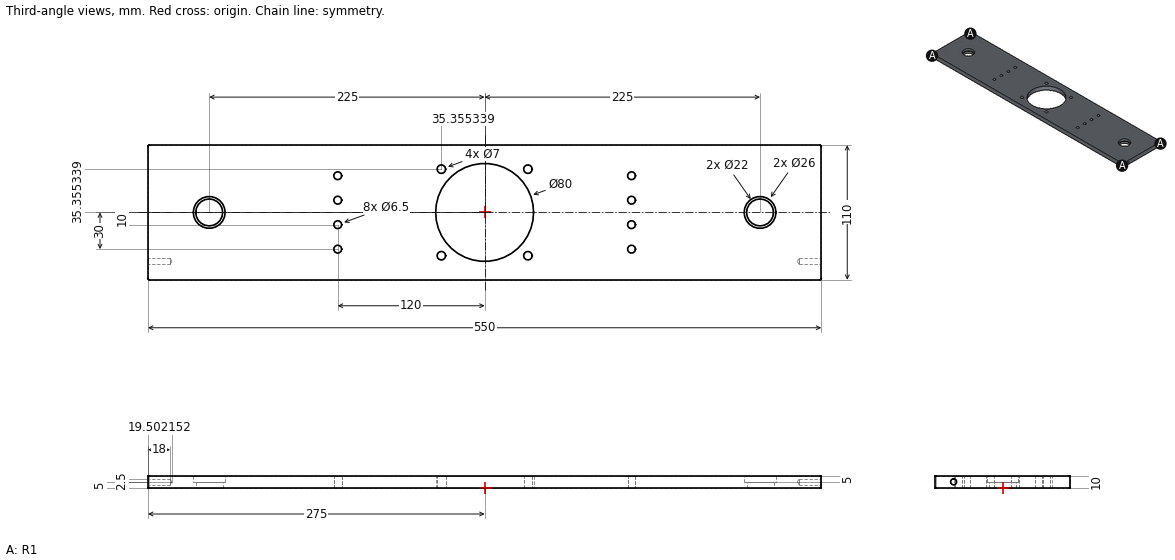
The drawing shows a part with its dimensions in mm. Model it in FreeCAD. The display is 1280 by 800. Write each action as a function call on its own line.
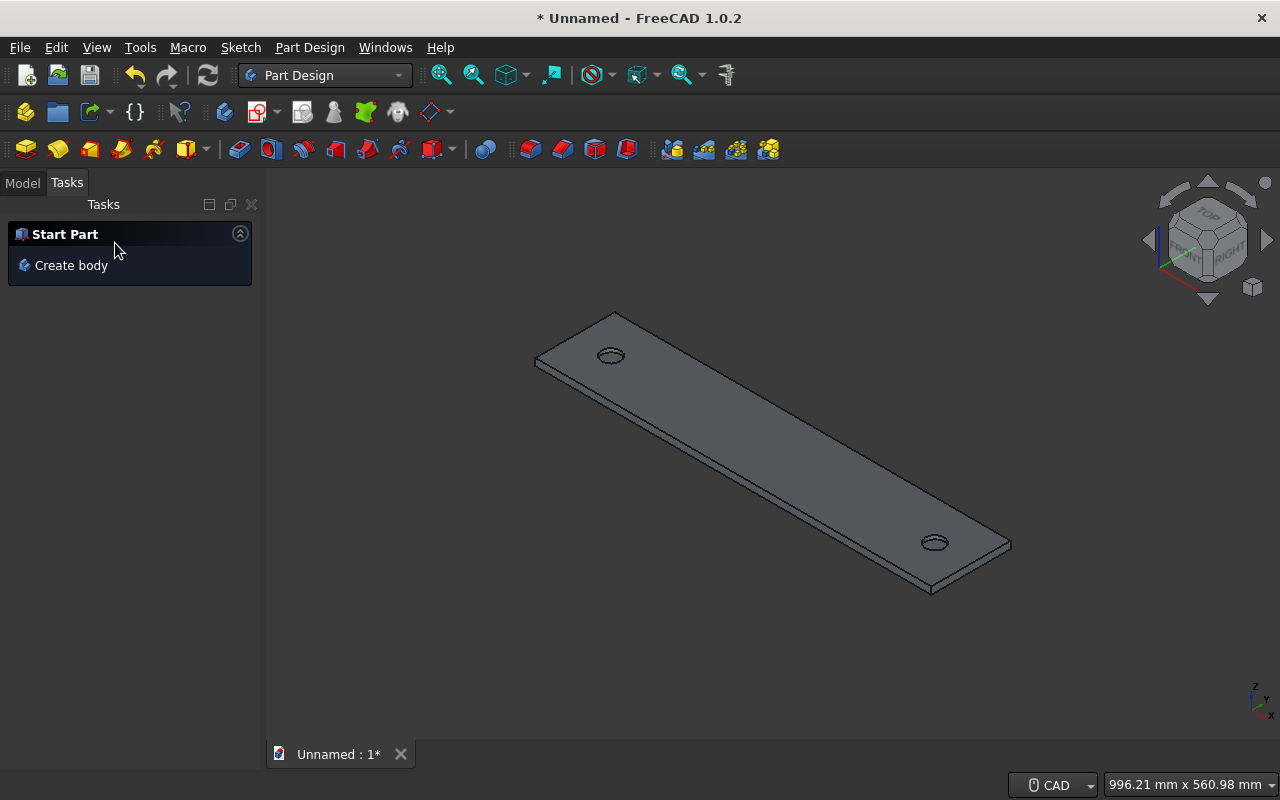
key(2)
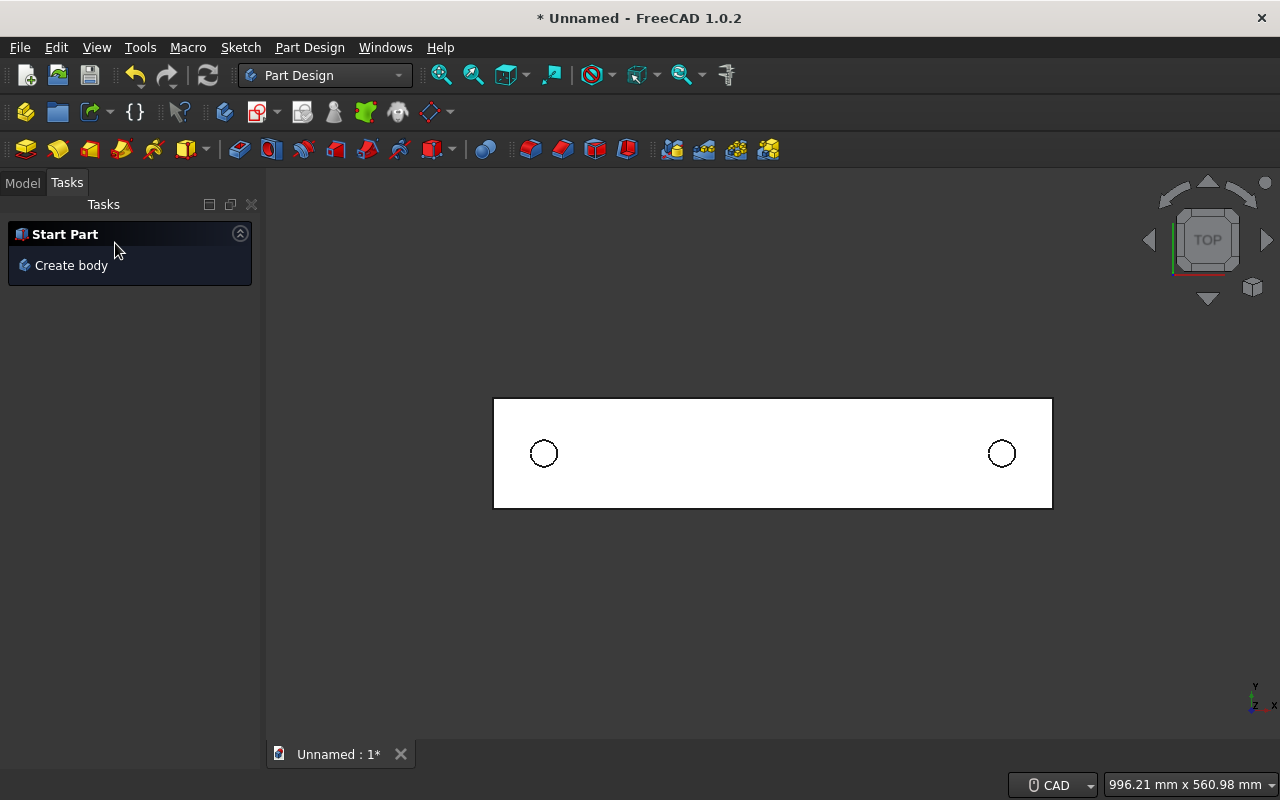
click(544, 452)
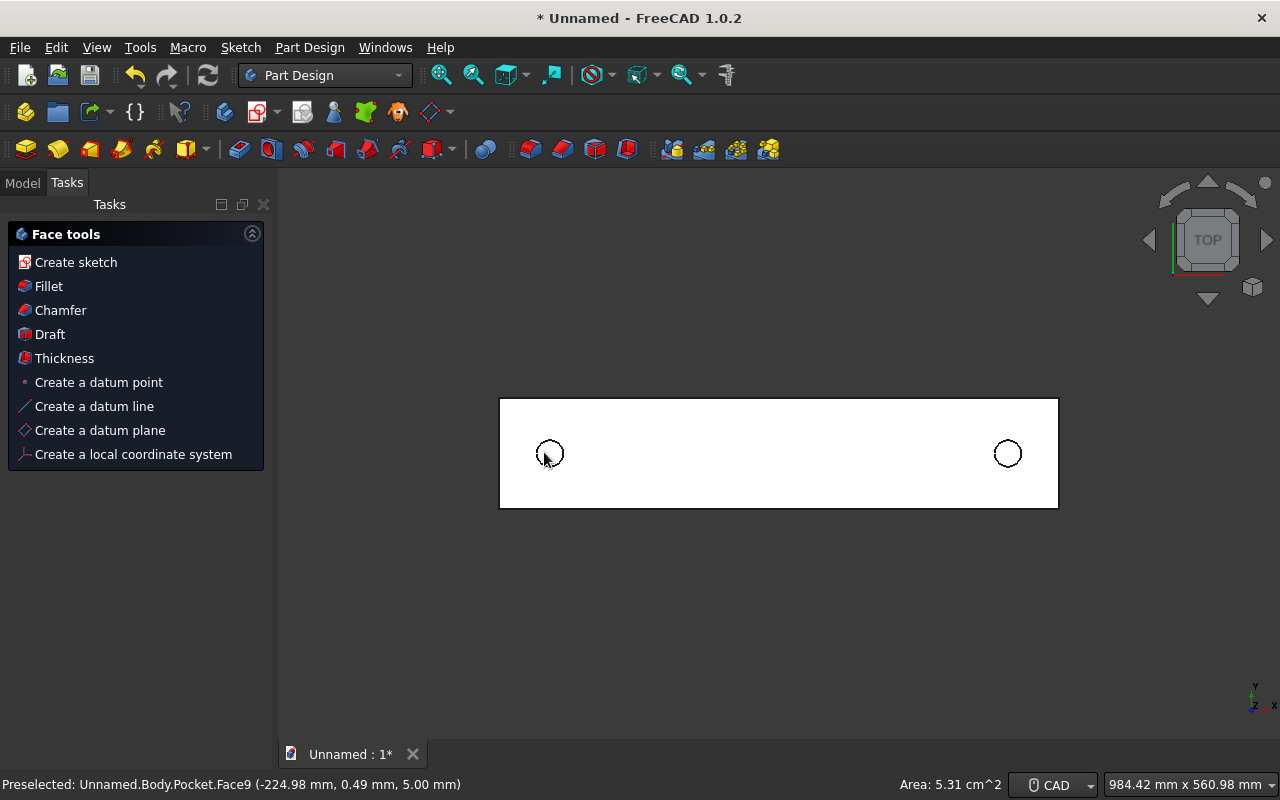
click(258, 112)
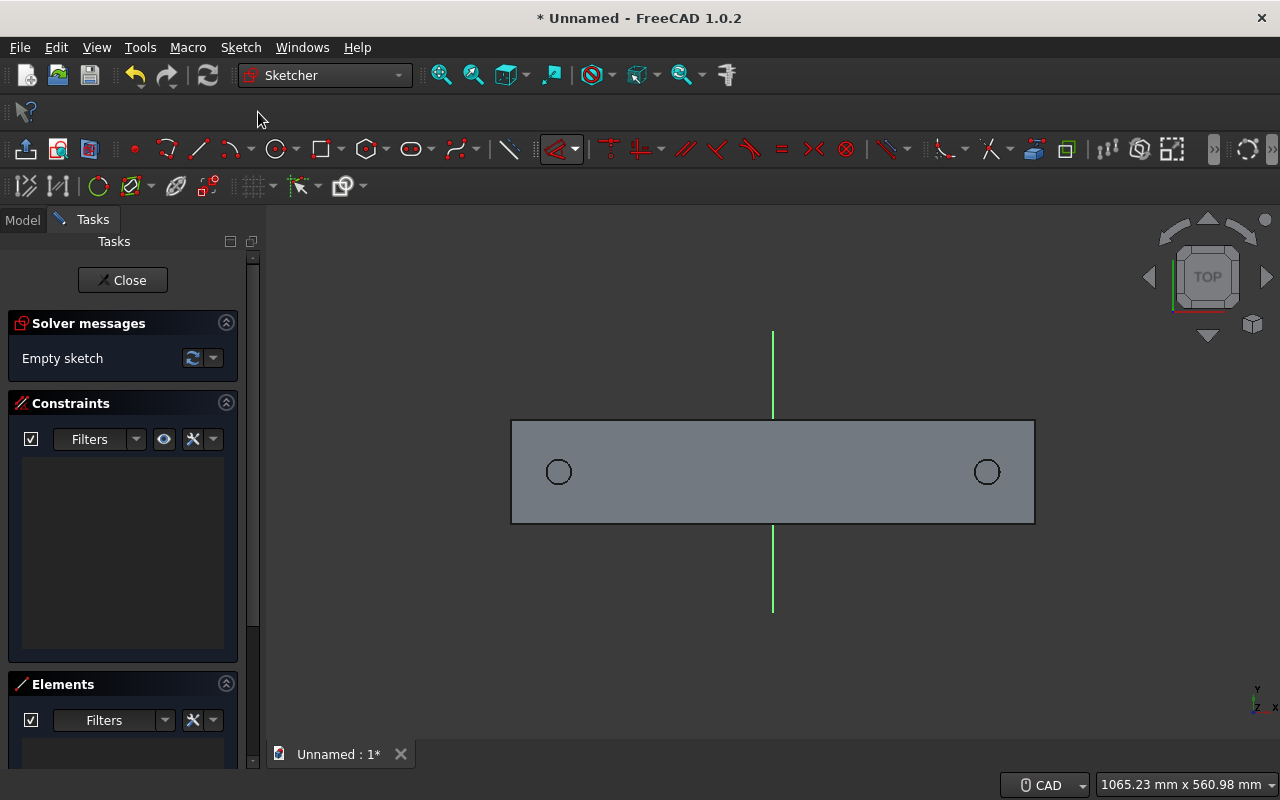
key(q)
key(s)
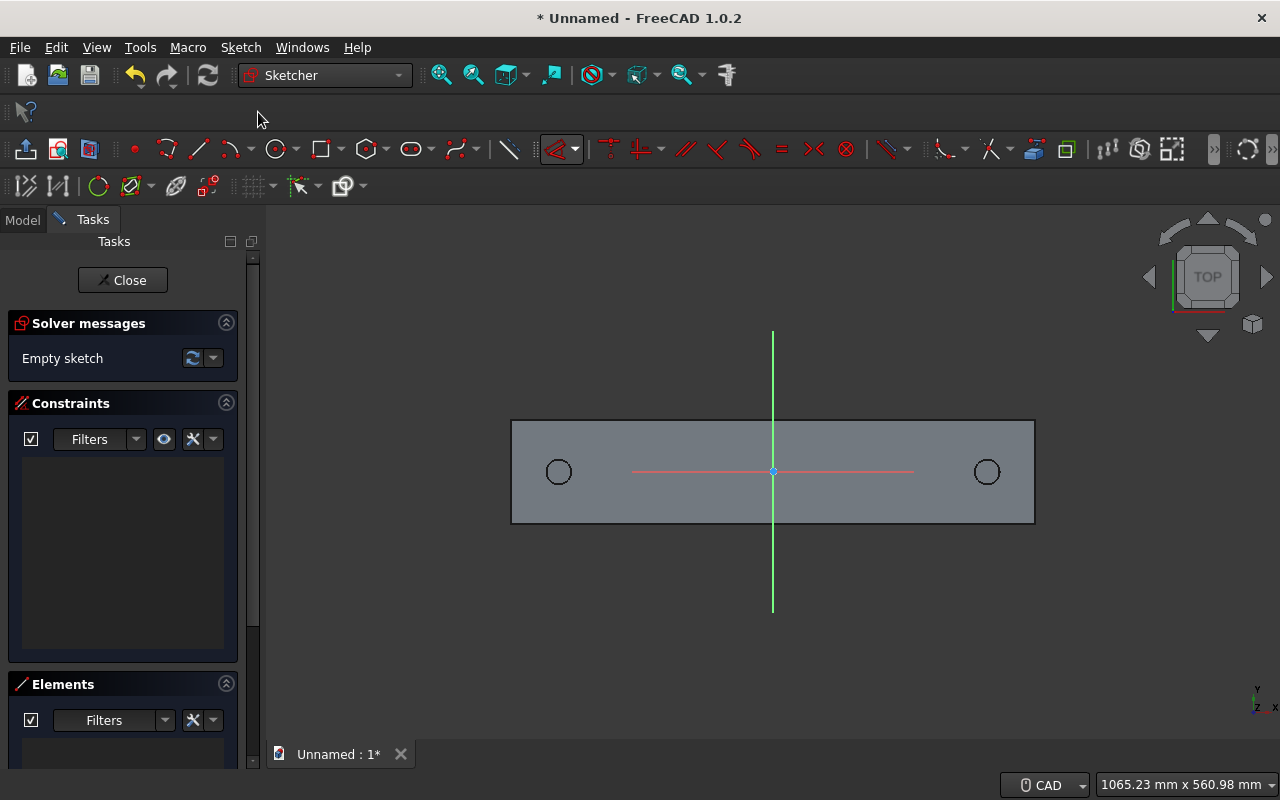
key(g)
key(c)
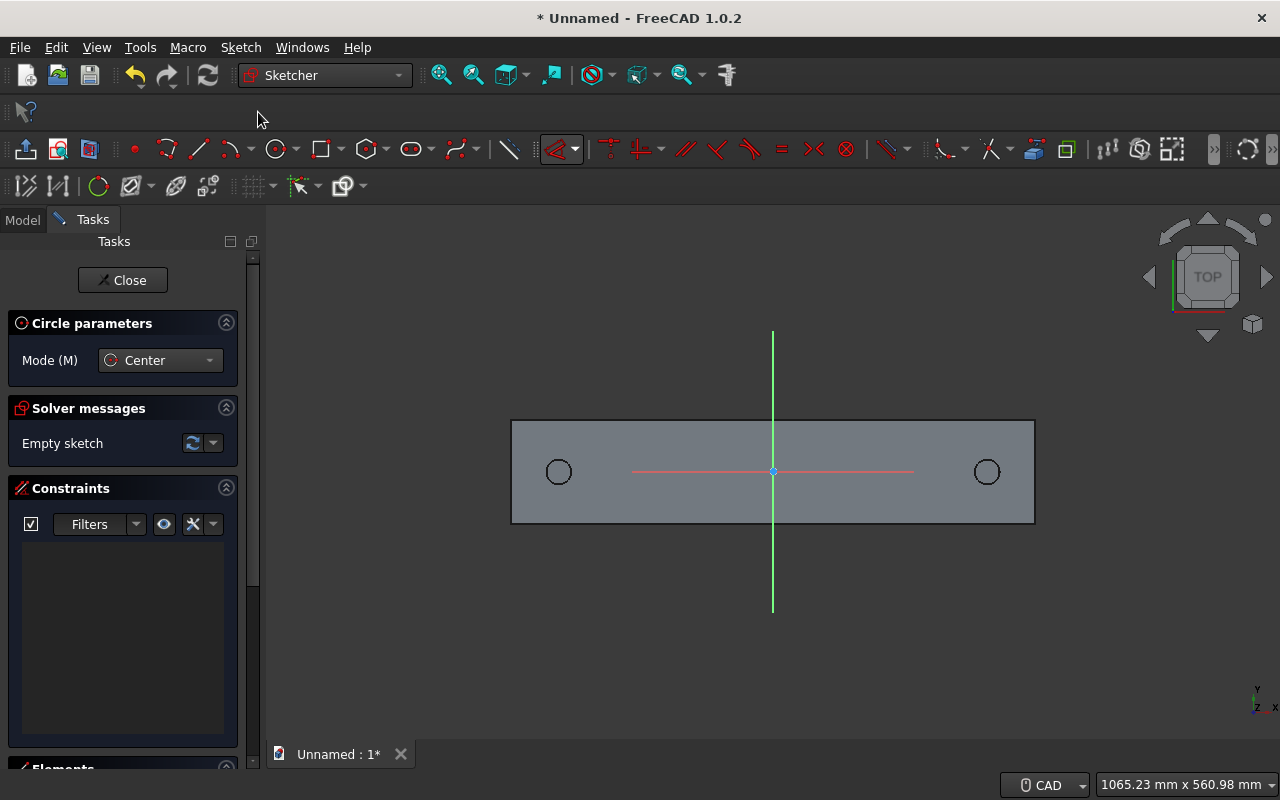
scroll(987, 472, up, 4)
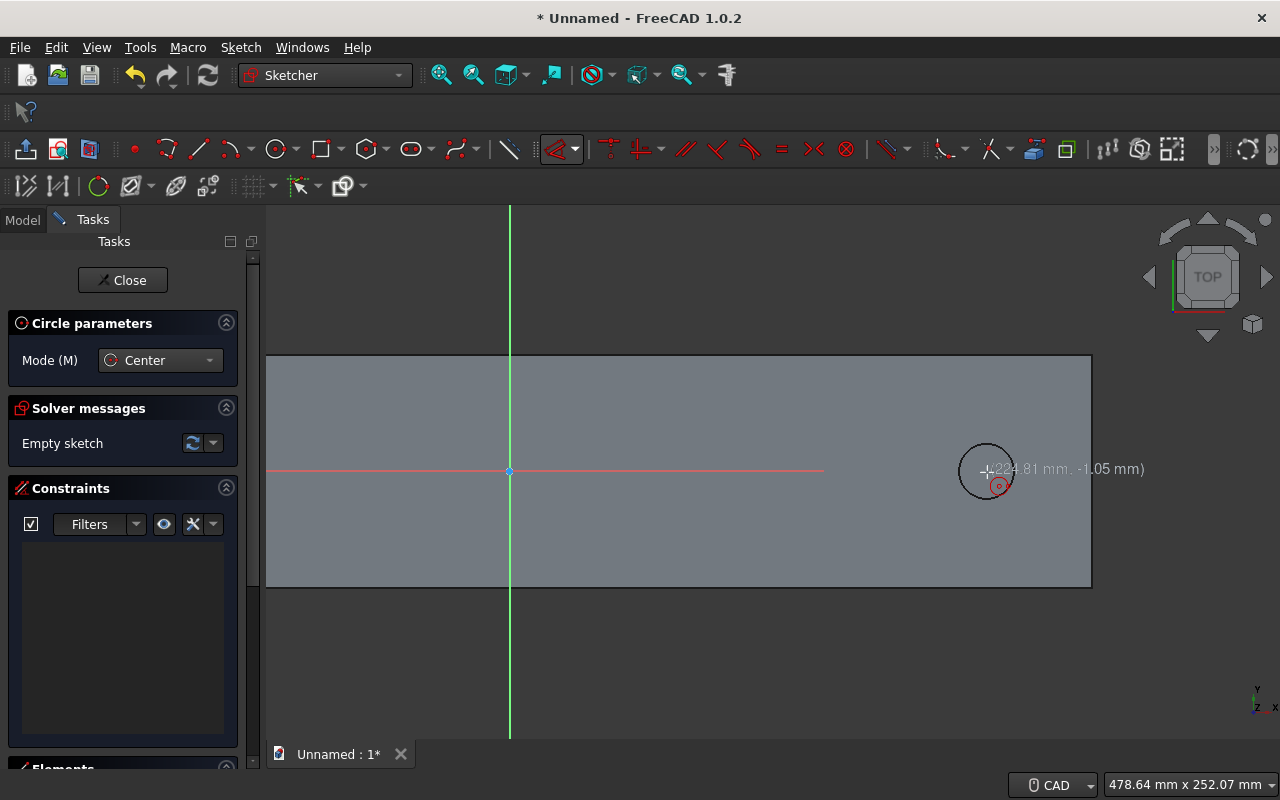
click(987, 471)
move(1003, 455)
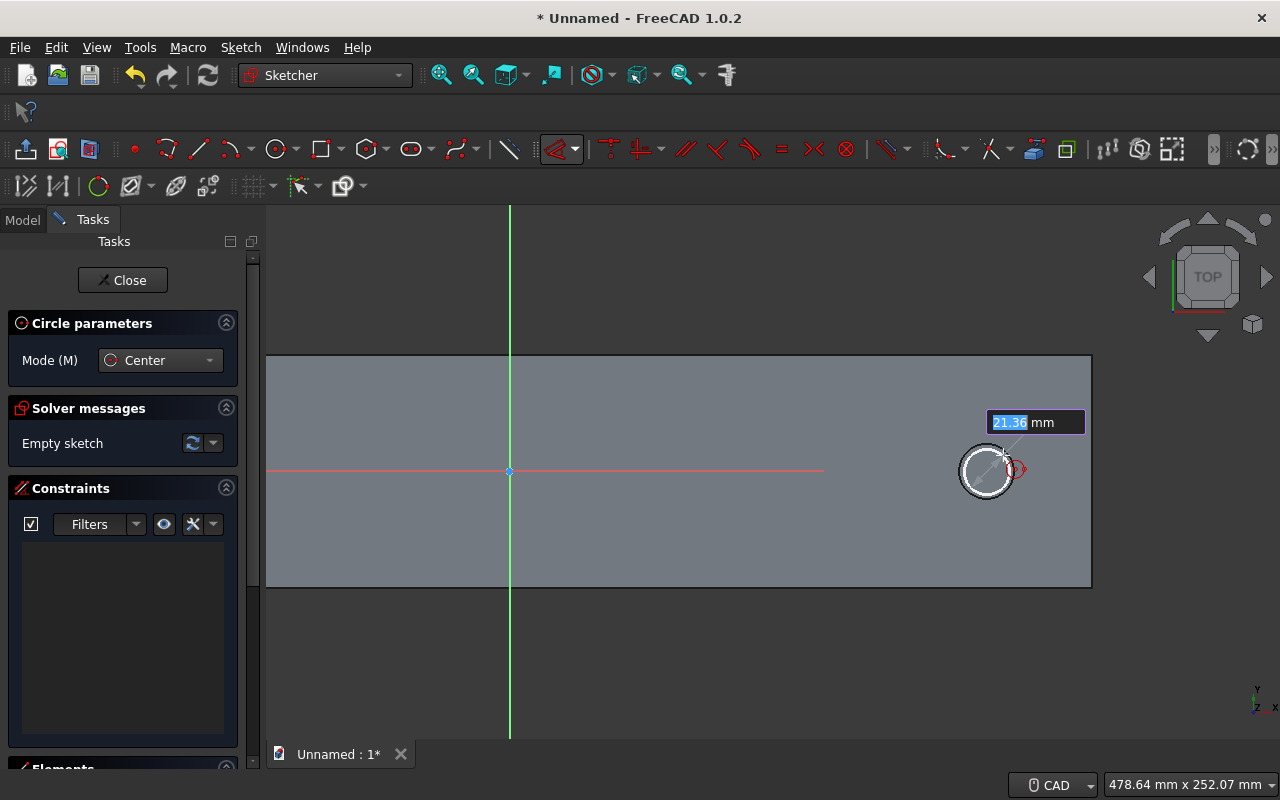
text(22)
key(Return)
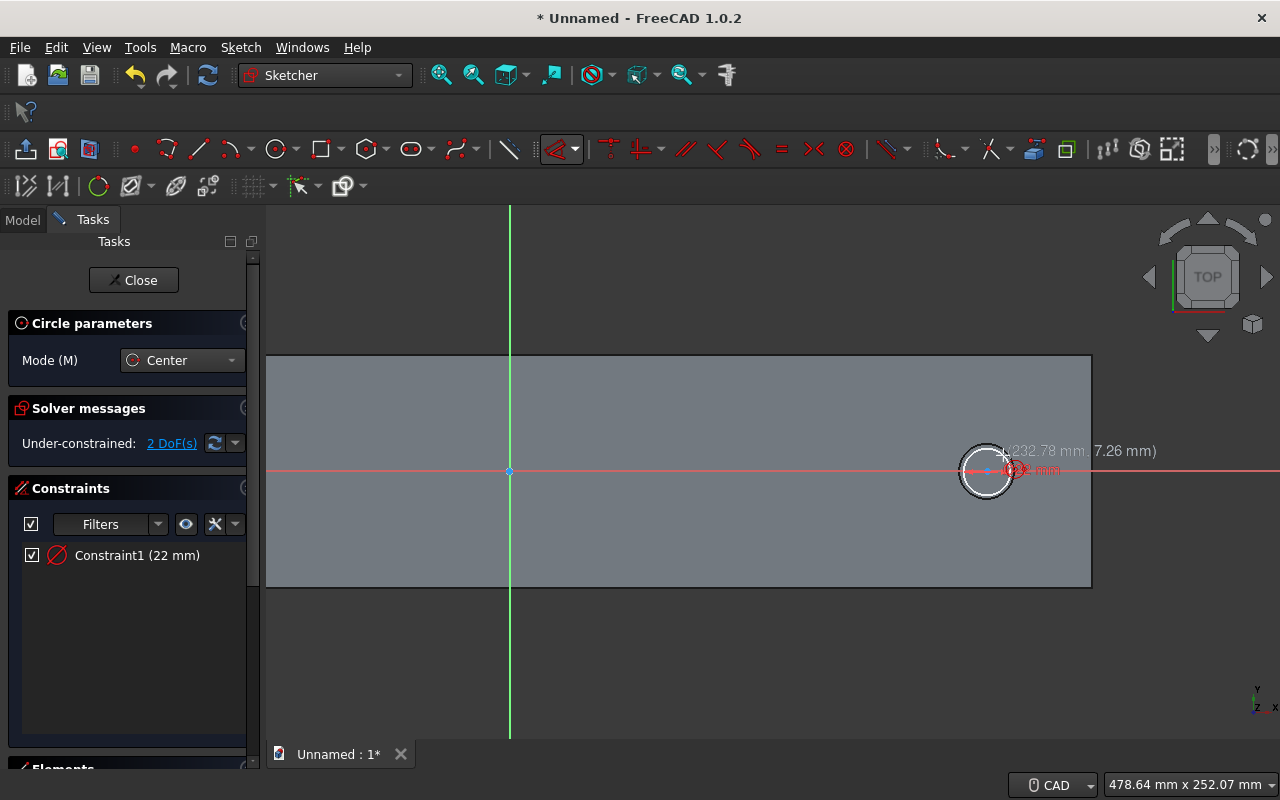
scroll(941, 473, down, 3)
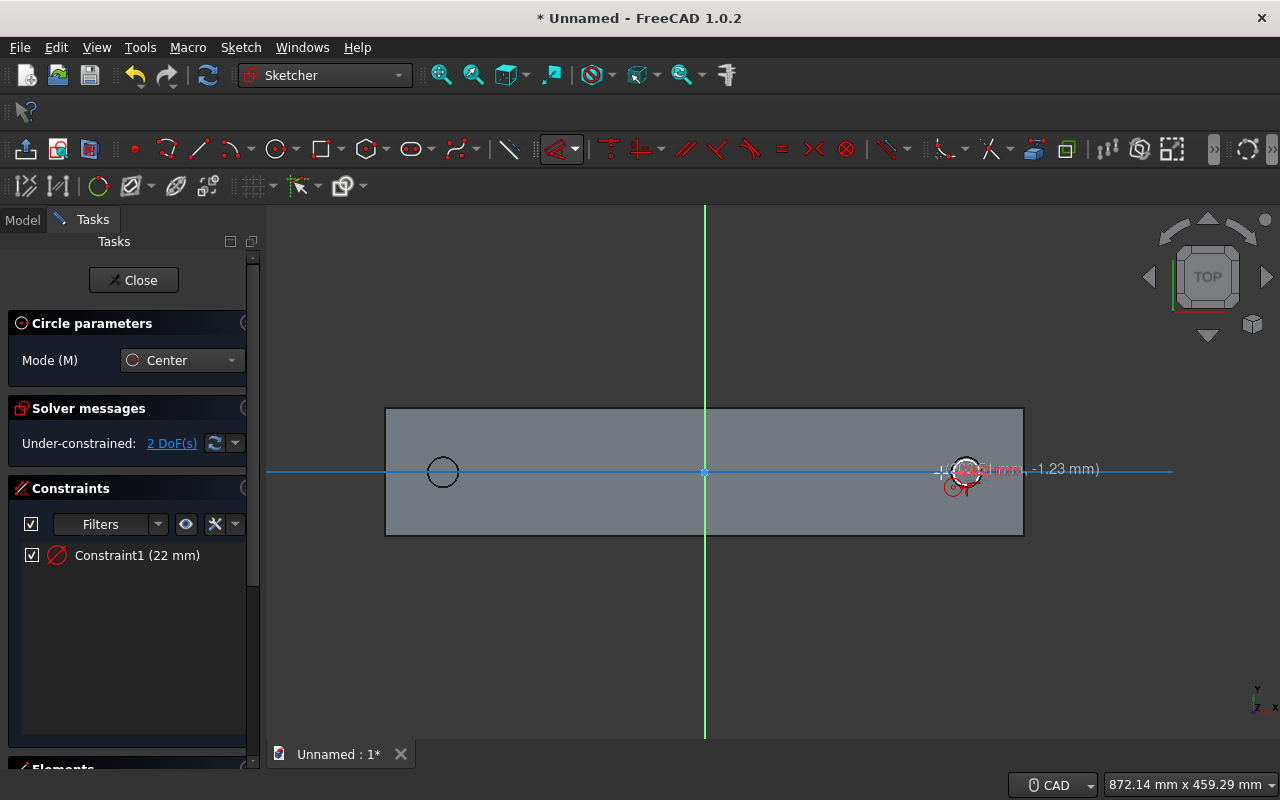
scroll(443, 472, up, 3)